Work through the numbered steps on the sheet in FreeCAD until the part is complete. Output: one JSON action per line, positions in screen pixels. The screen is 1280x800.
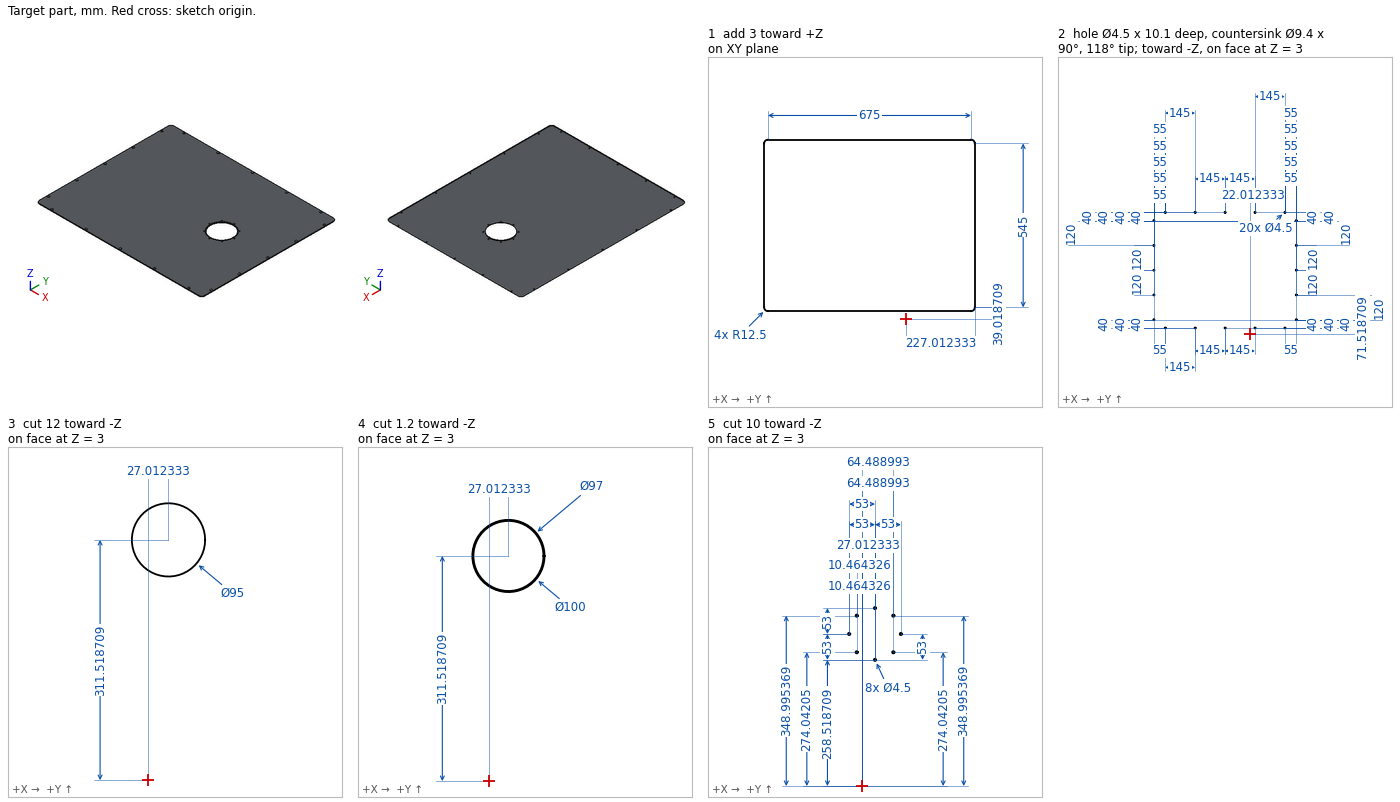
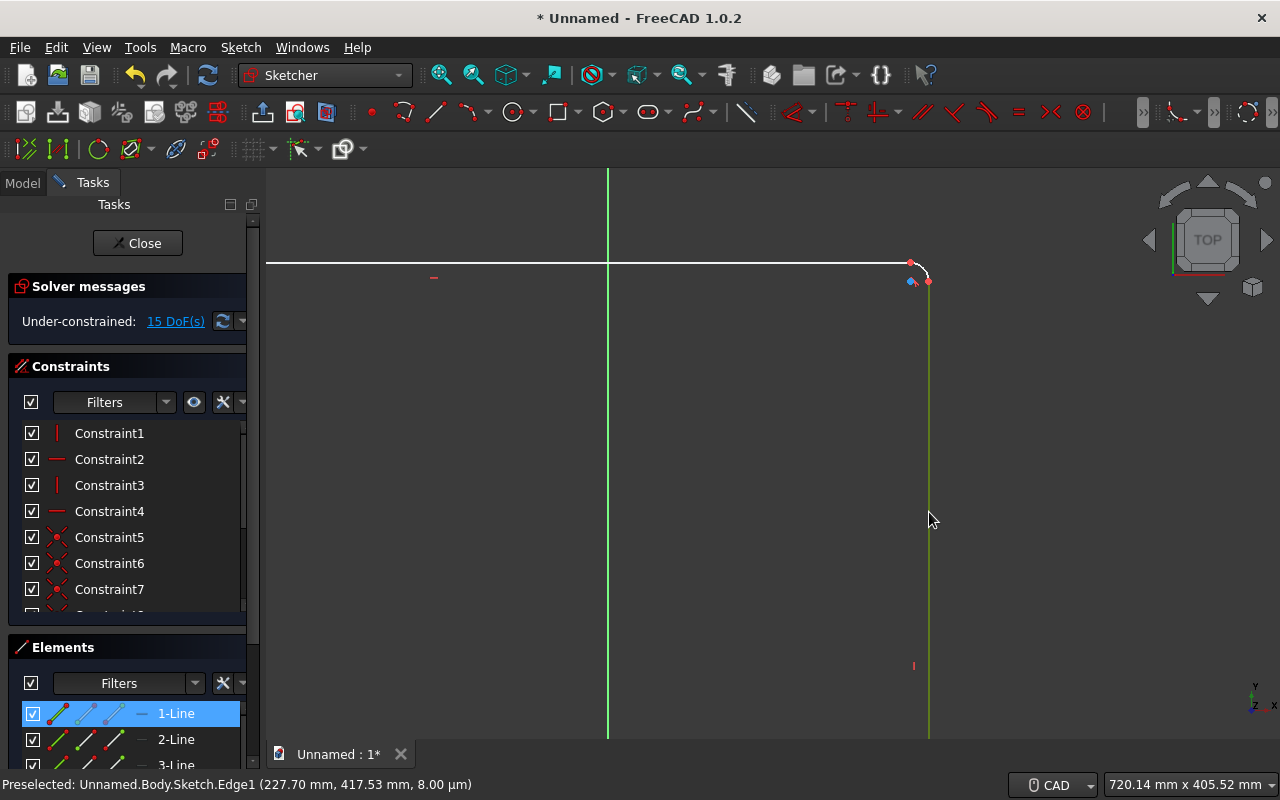
{"action": "scroll", "coordinate": [924, 268], "scroll_direction": "down", "scroll_amount": 4}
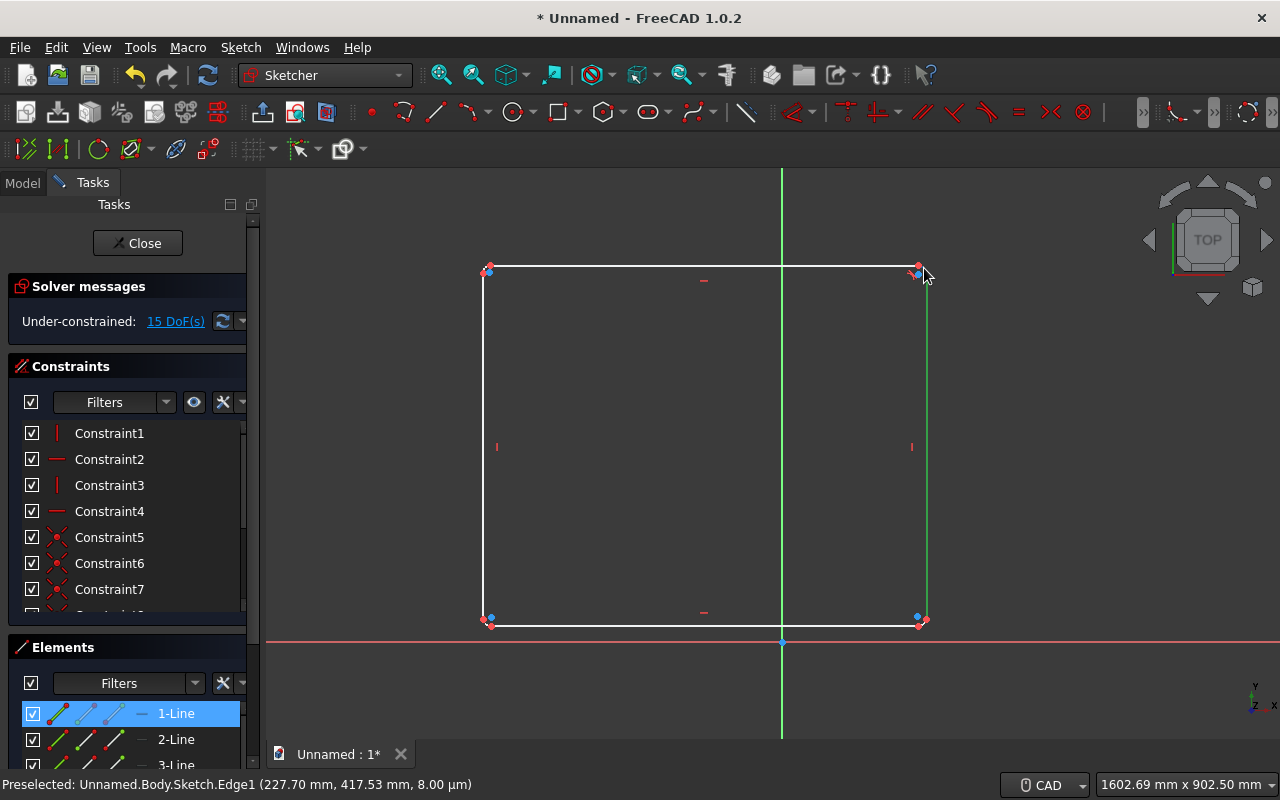
{"action": "scroll", "coordinate": [924, 624], "scroll_direction": "up", "scroll_amount": 5}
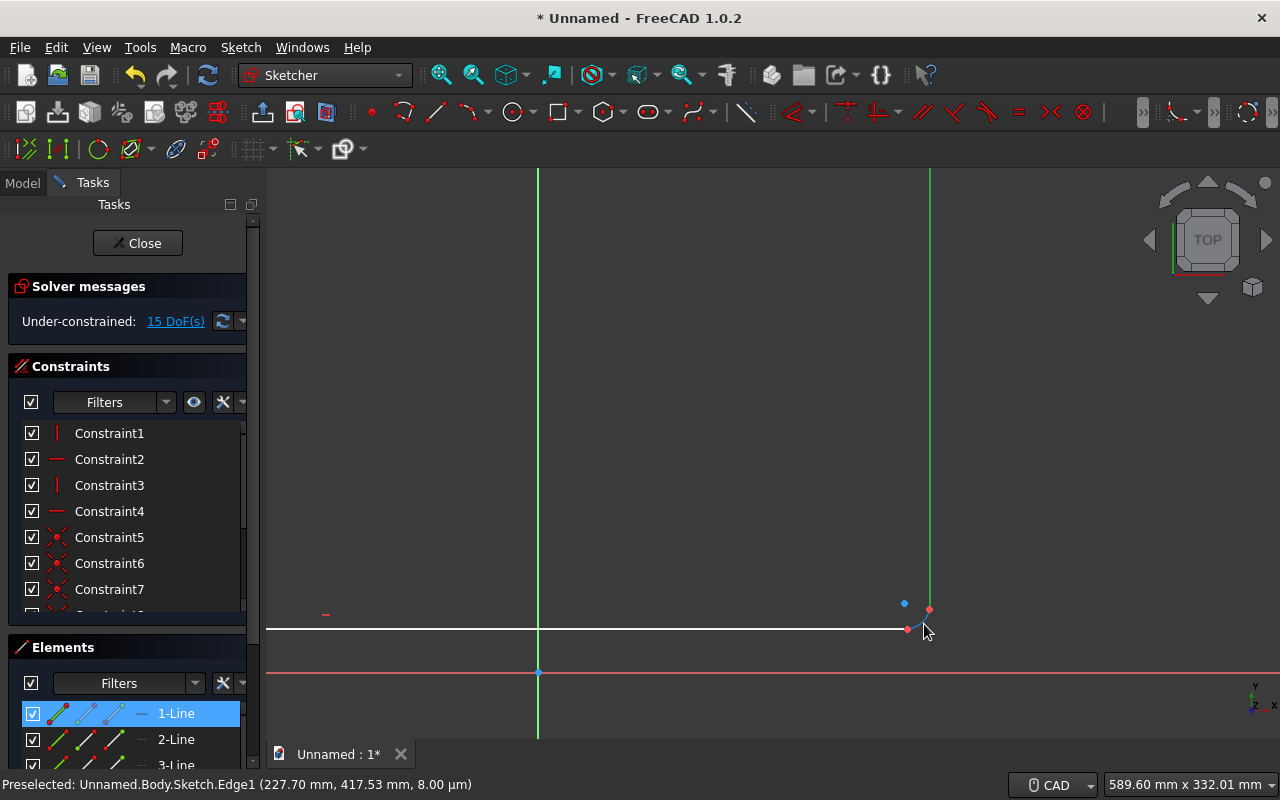
{"action": "left_click", "coordinate": [922, 623]}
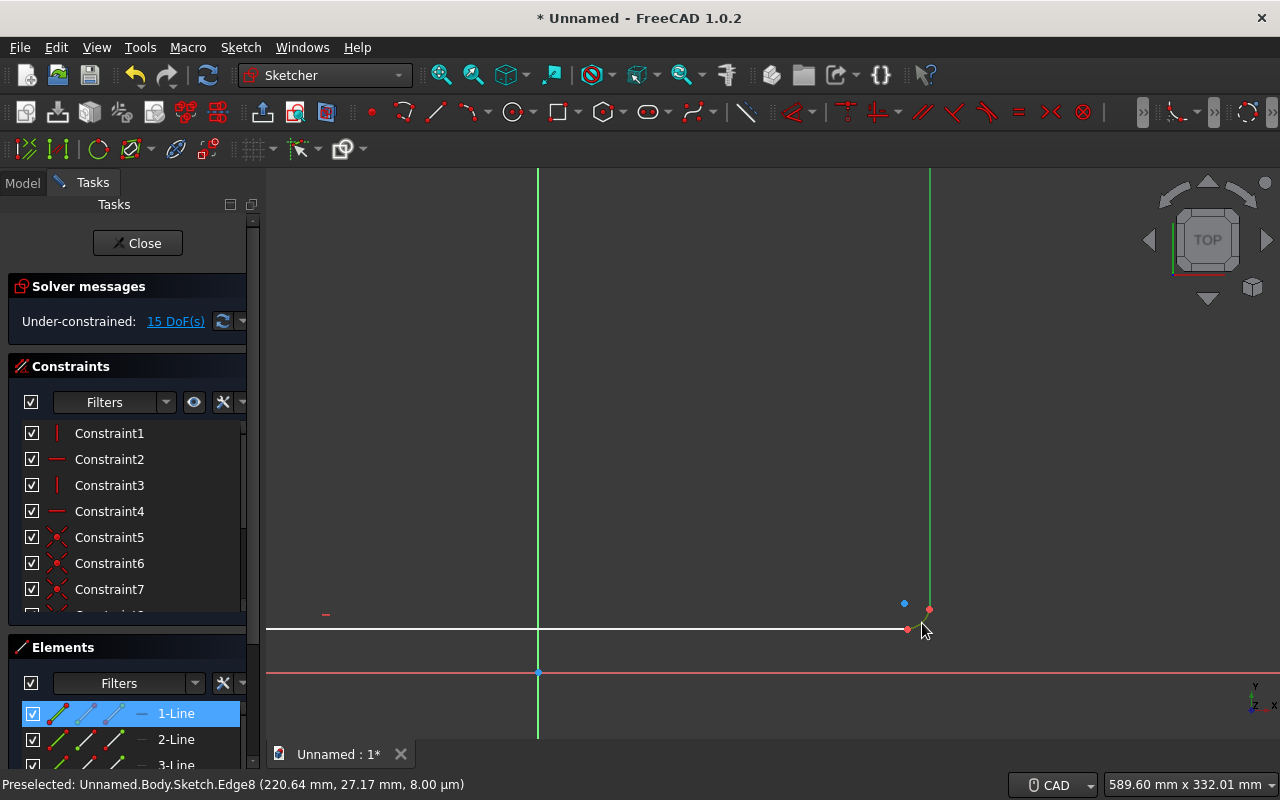
{"action": "left_click", "coordinate": [988, 112]}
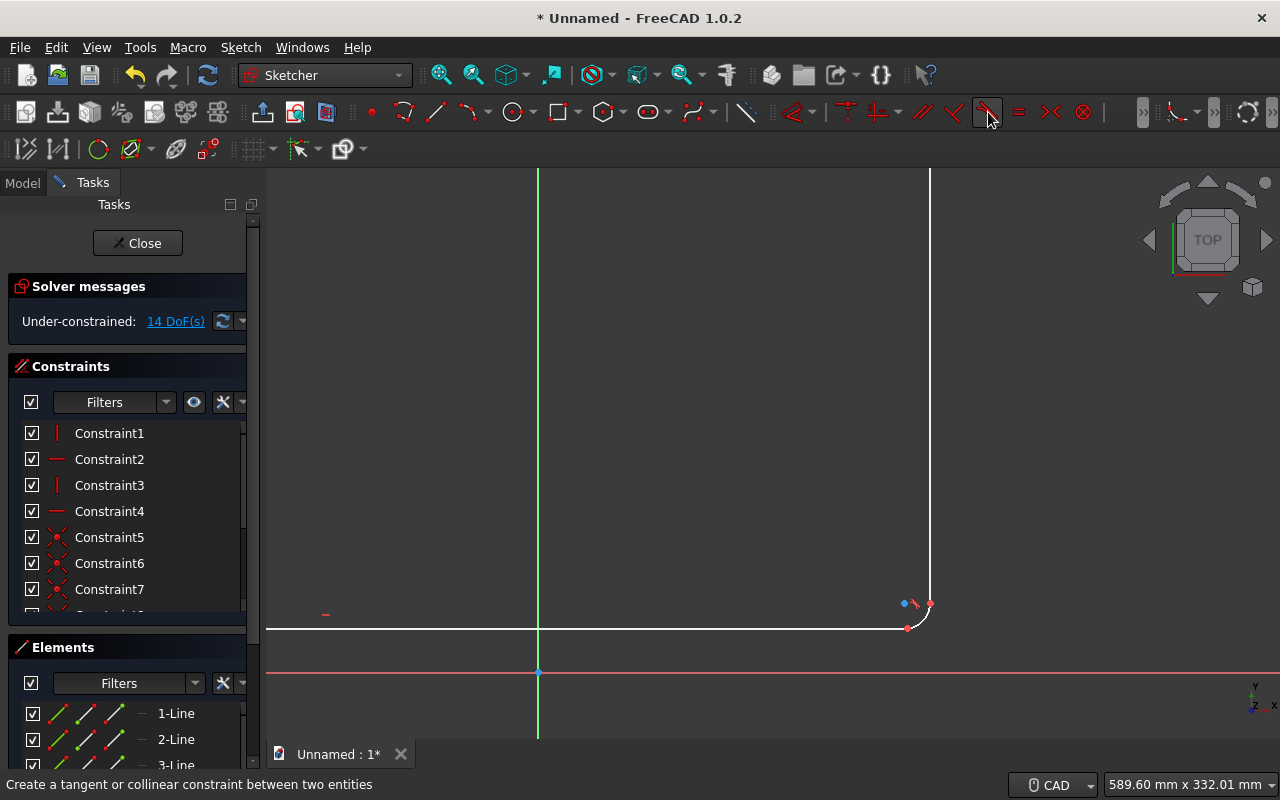
{"action": "scroll", "coordinate": [924, 625], "scroll_direction": "down", "scroll_amount": 5}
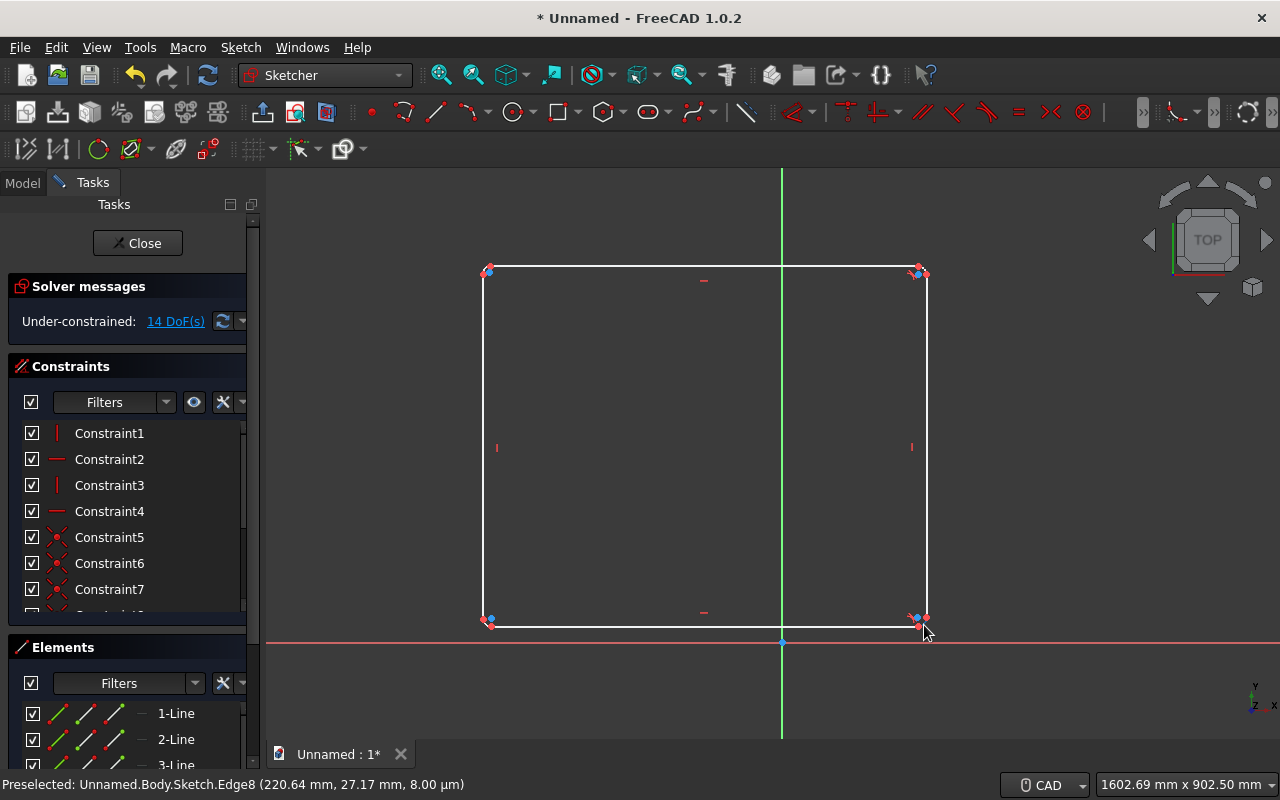
{"action": "scroll", "coordinate": [790, 266], "scroll_direction": "up", "scroll_amount": 3}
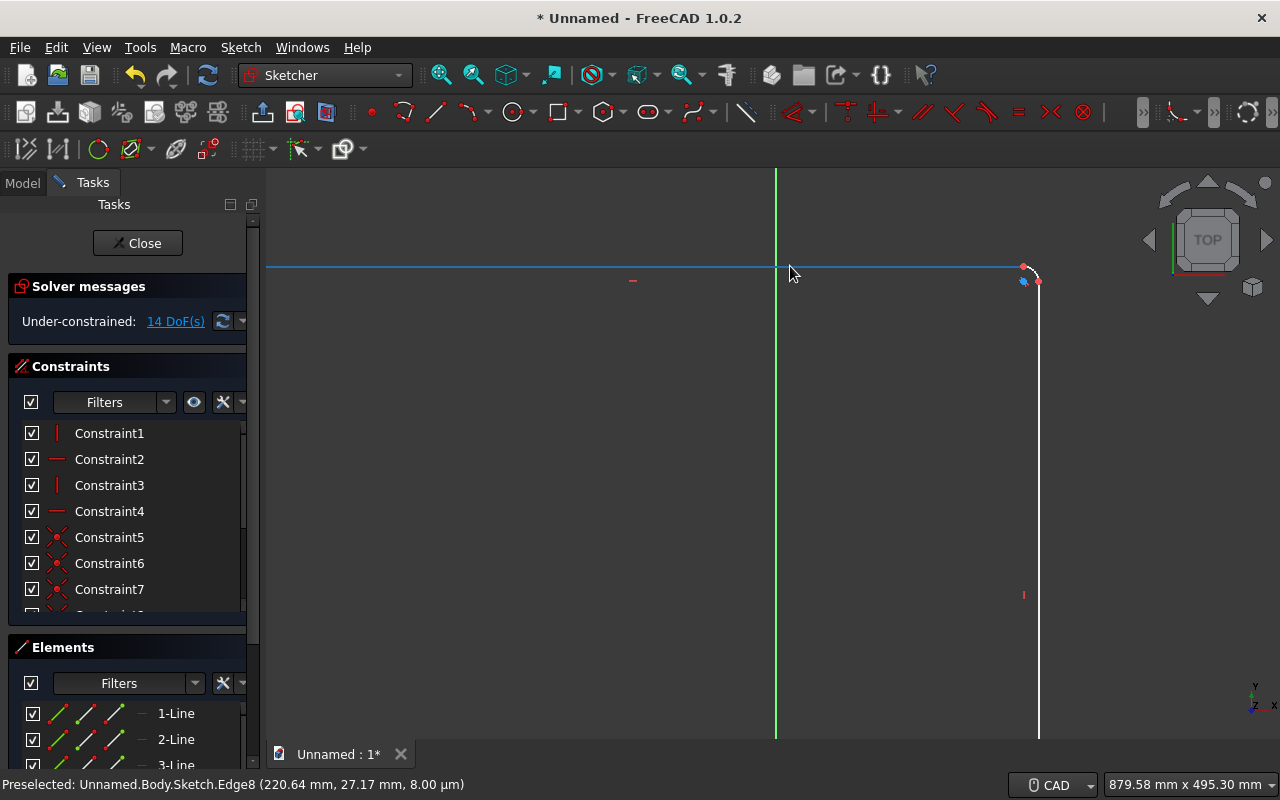
{"action": "left_click", "coordinate": [790, 267]}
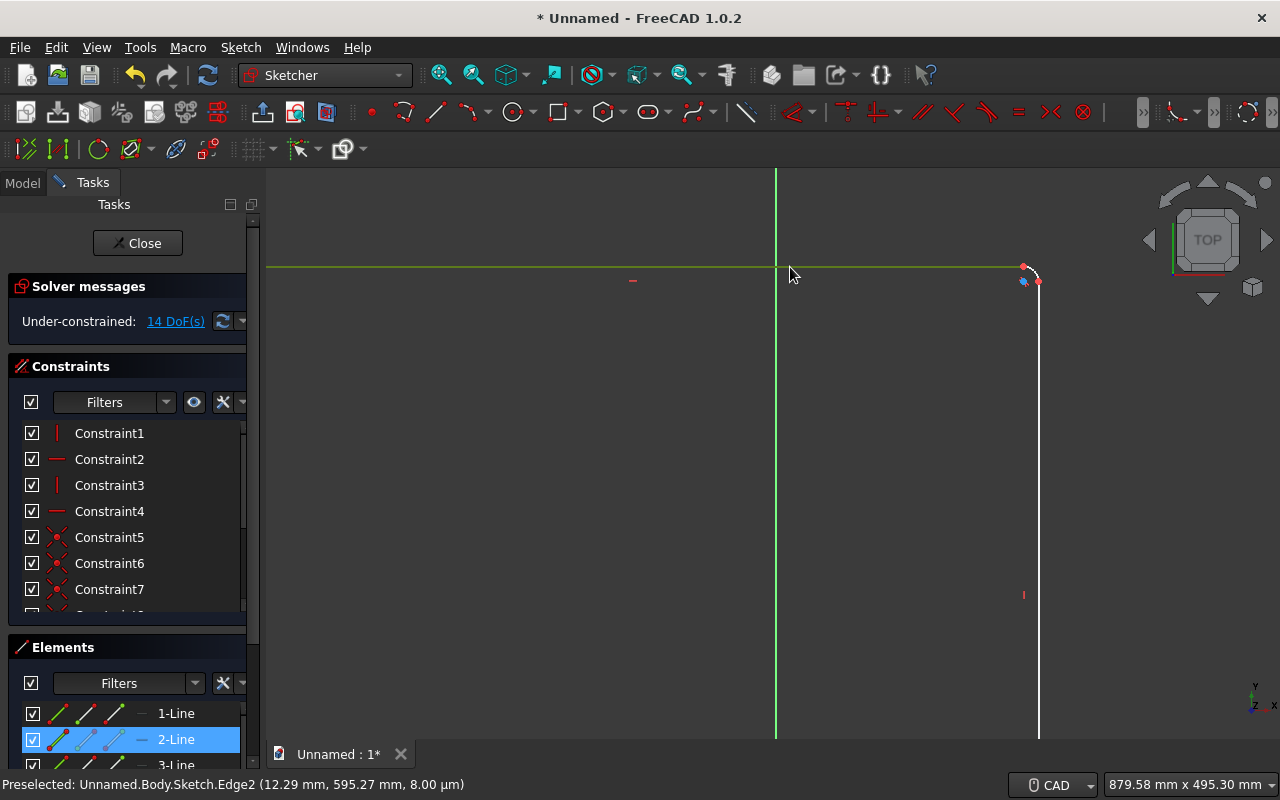
{"action": "left_click", "coordinate": [1034, 271]}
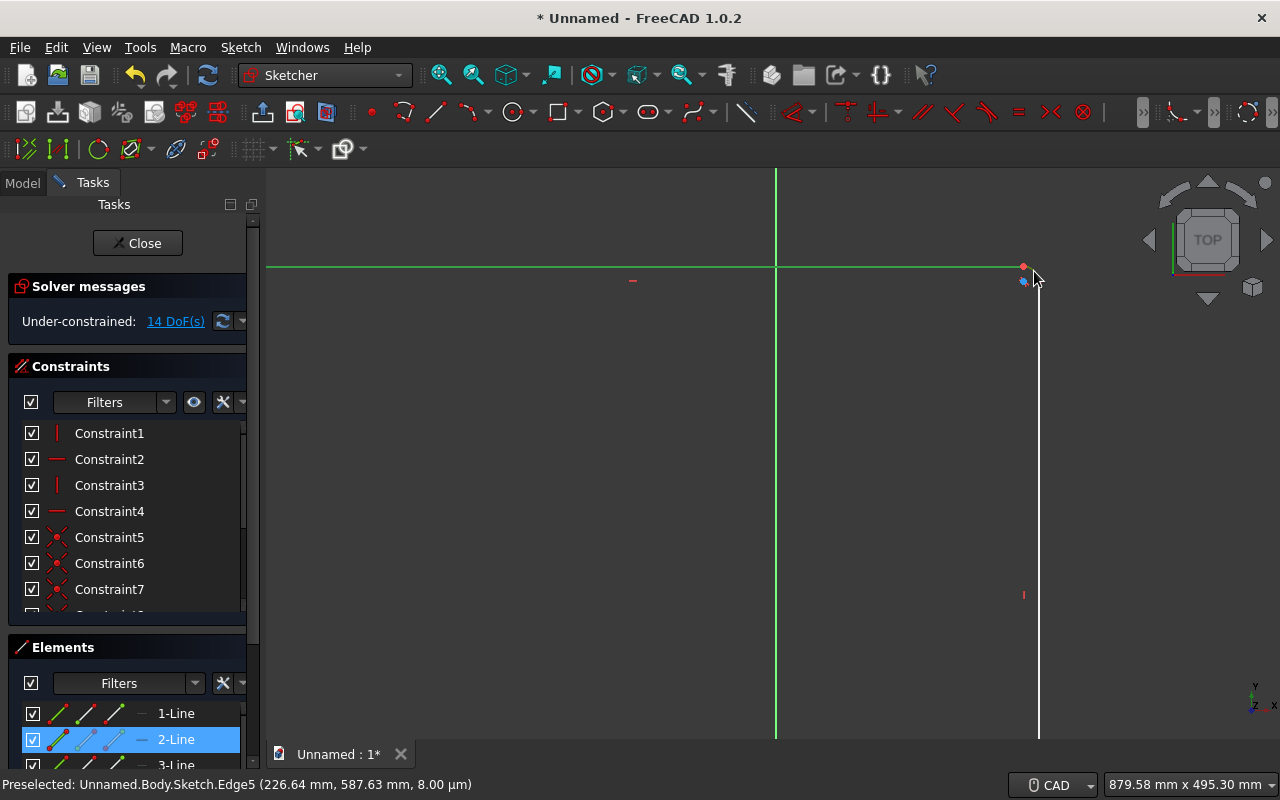
{"action": "left_click", "coordinate": [988, 112]}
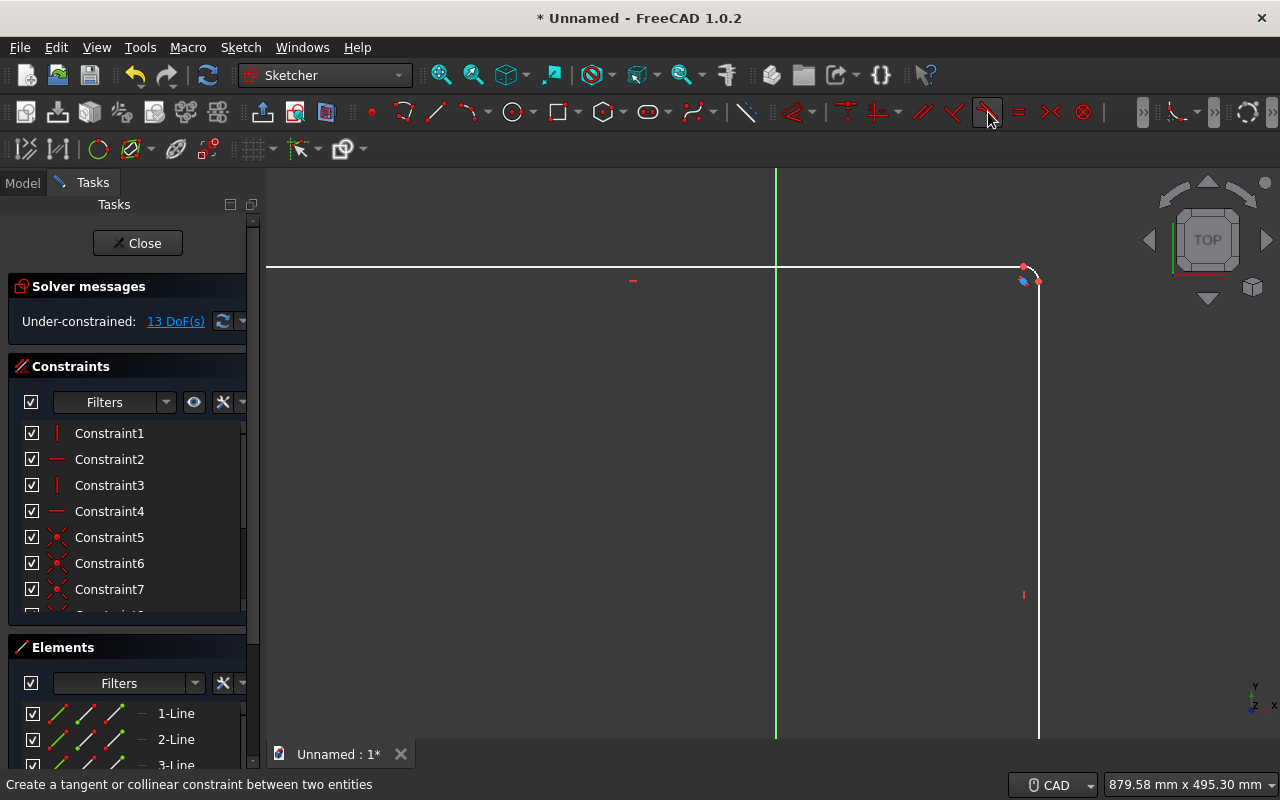
{"action": "left_click", "coordinate": [790, 267]}